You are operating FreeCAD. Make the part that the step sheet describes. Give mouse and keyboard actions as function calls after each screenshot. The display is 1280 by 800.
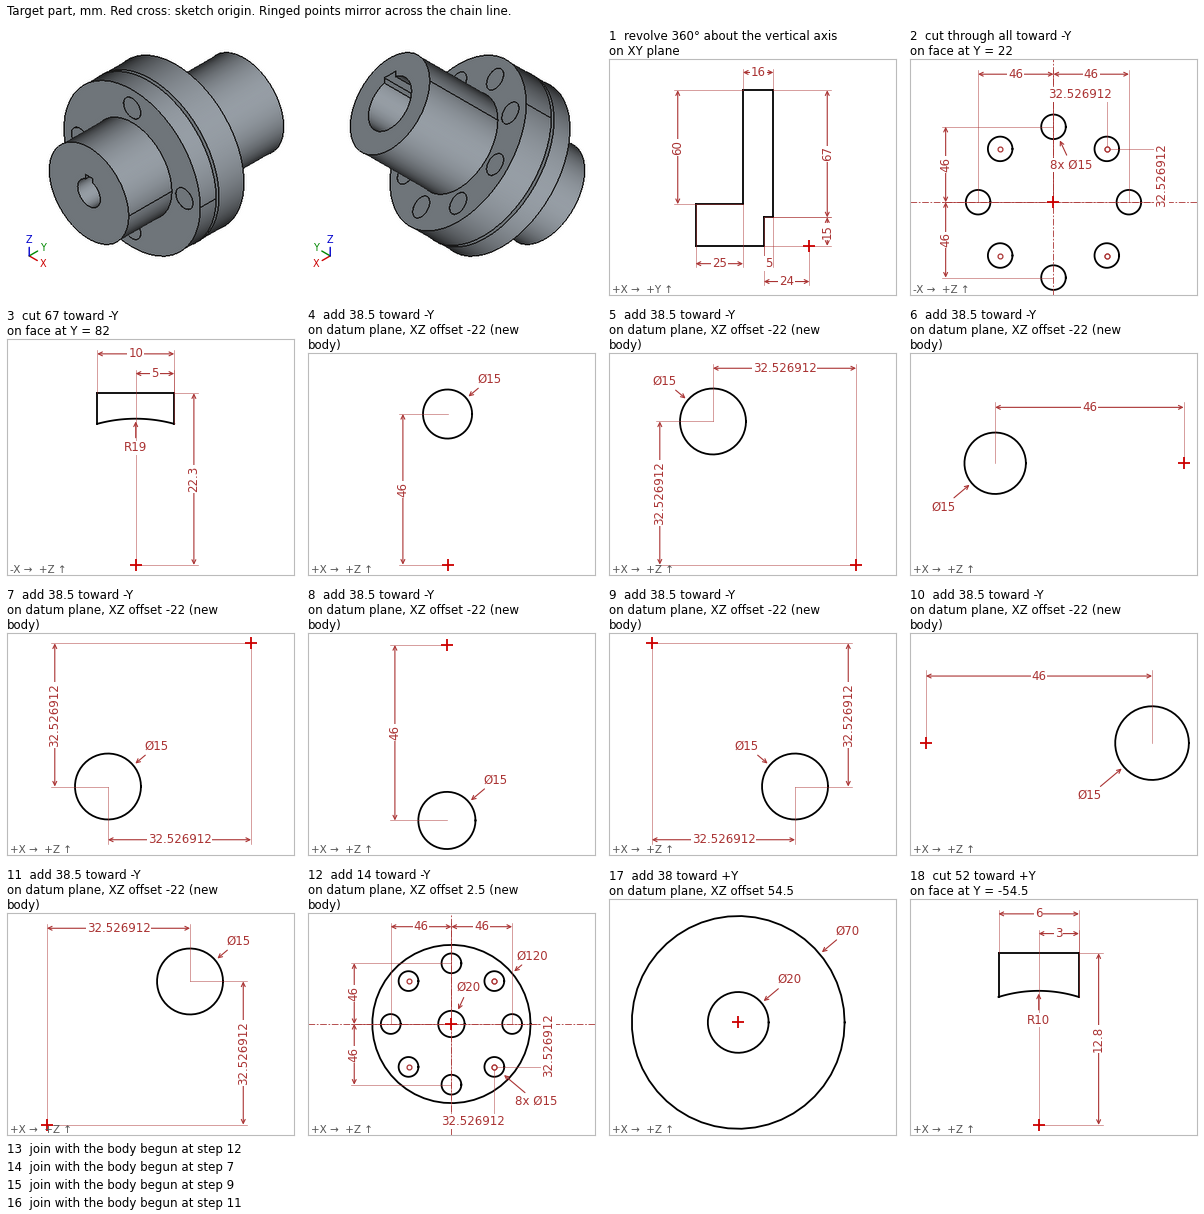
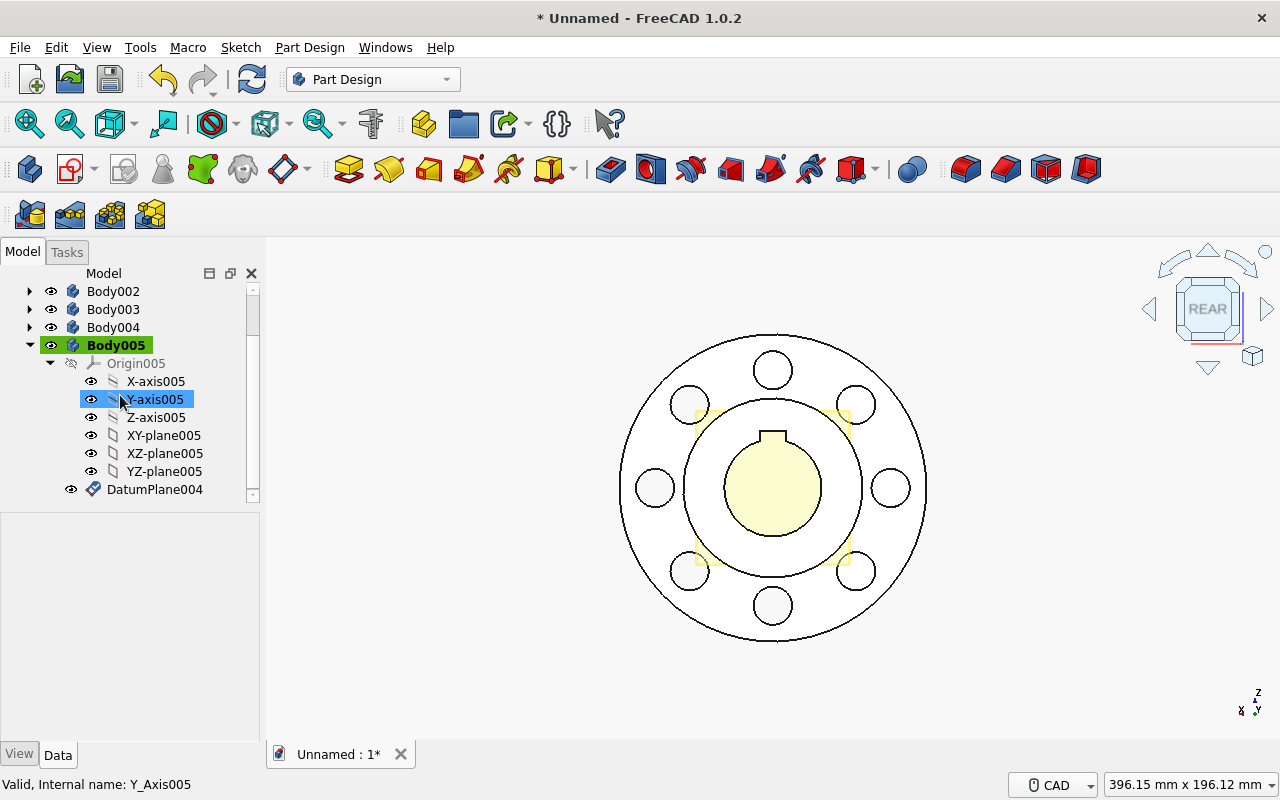
click(116, 489)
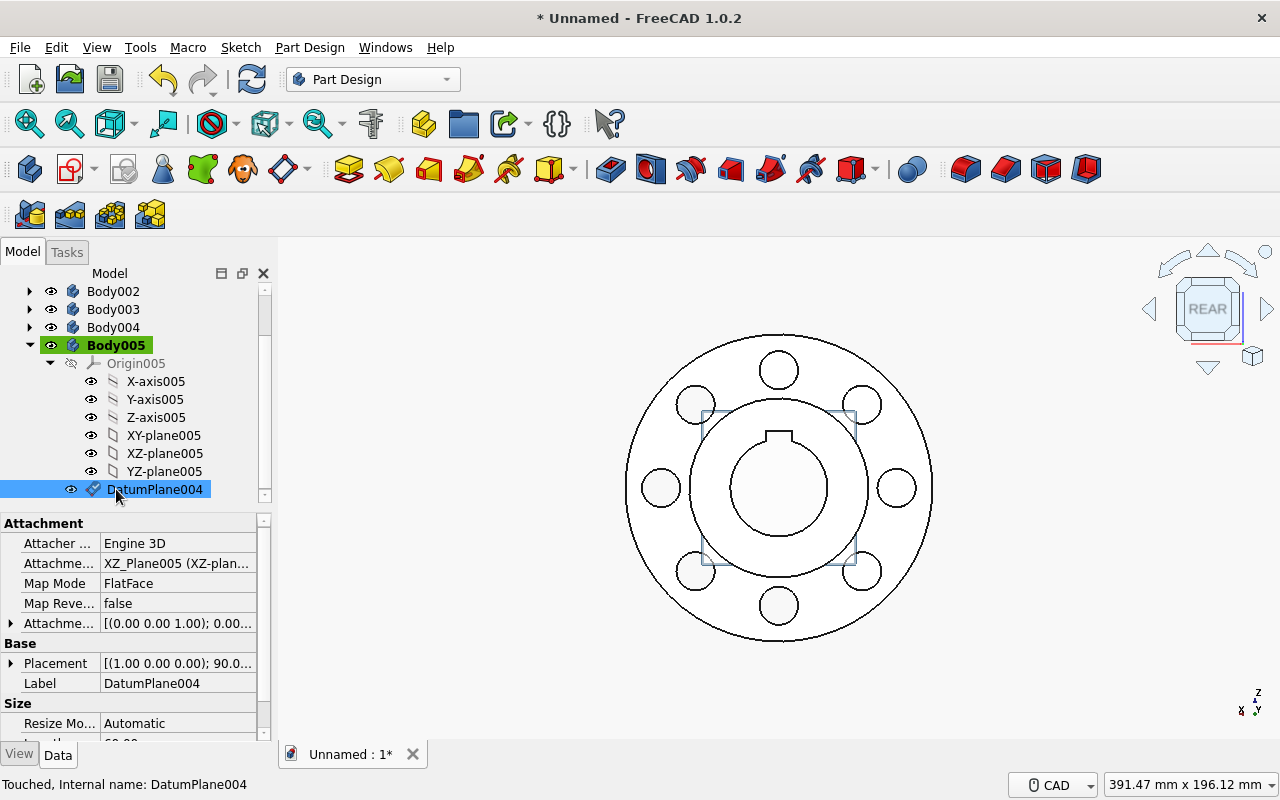
click(70, 170)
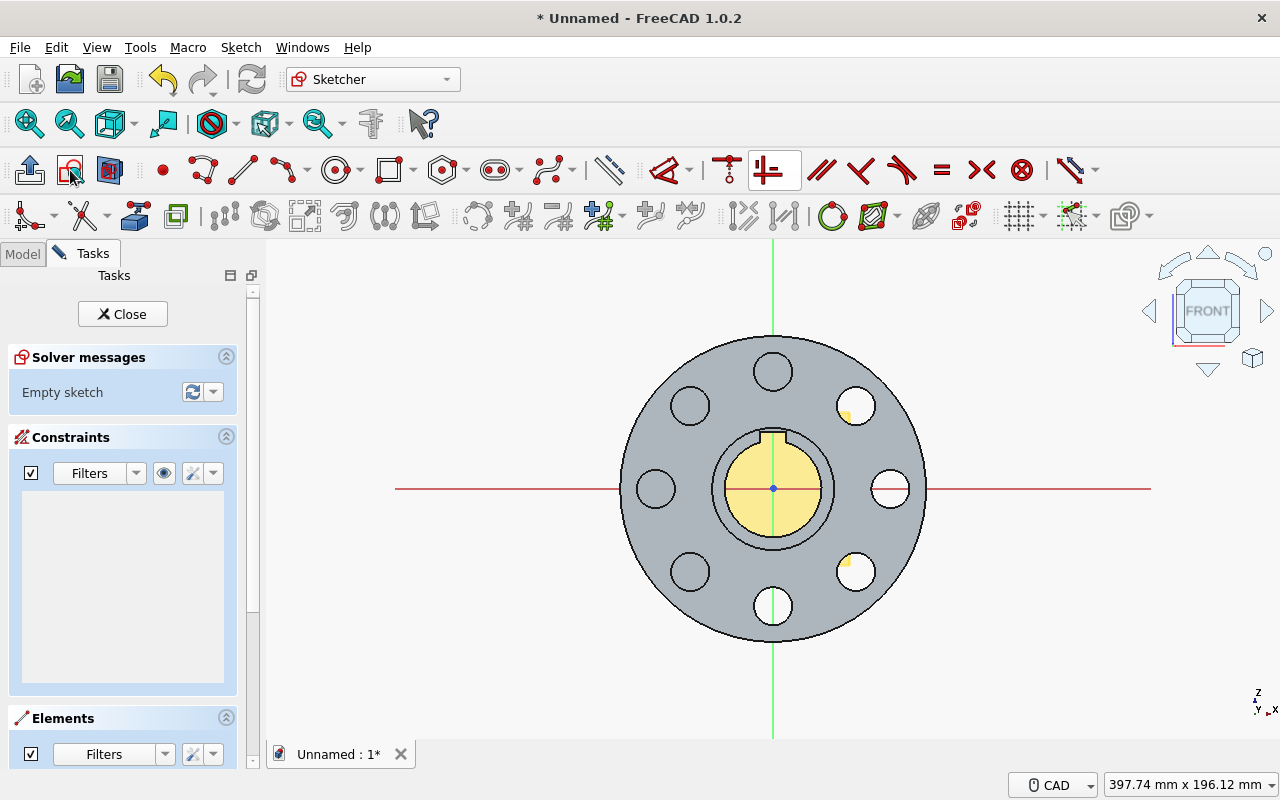
scroll(782, 621, up, 11)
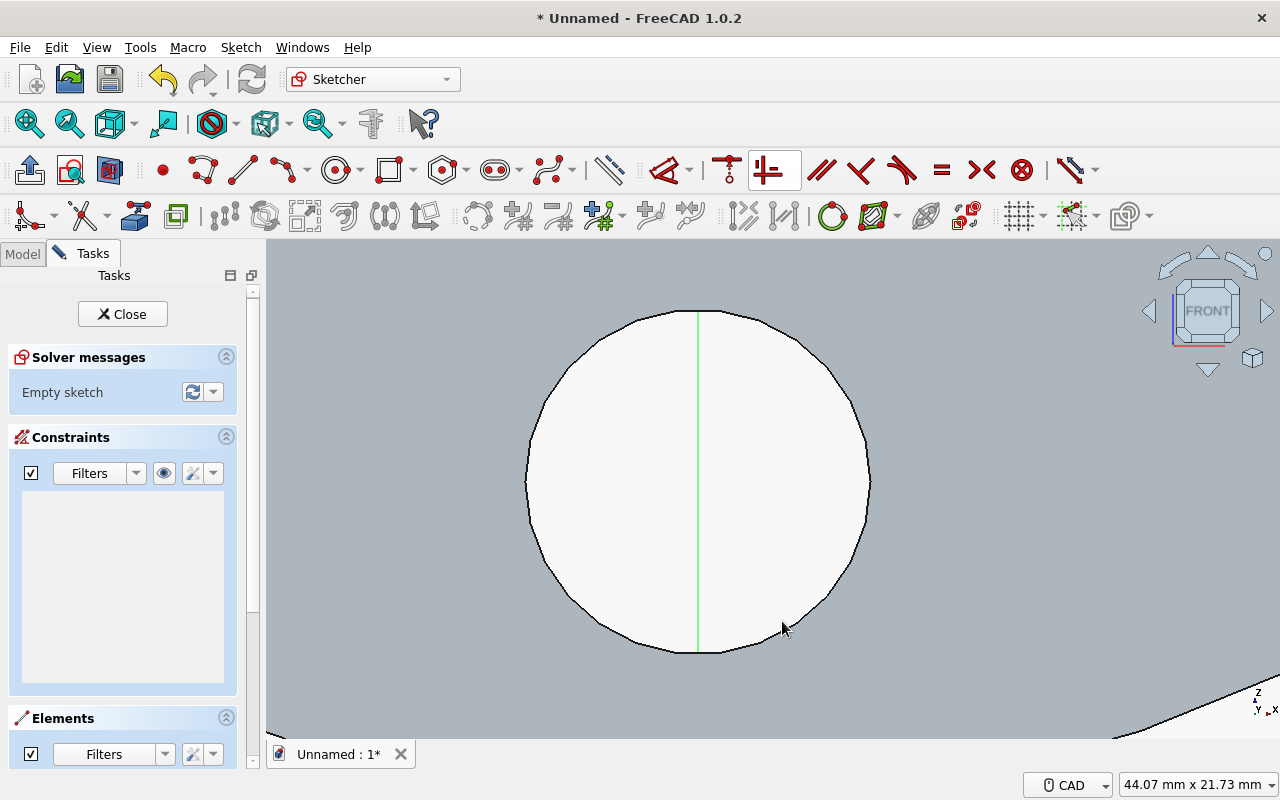
click(336, 170)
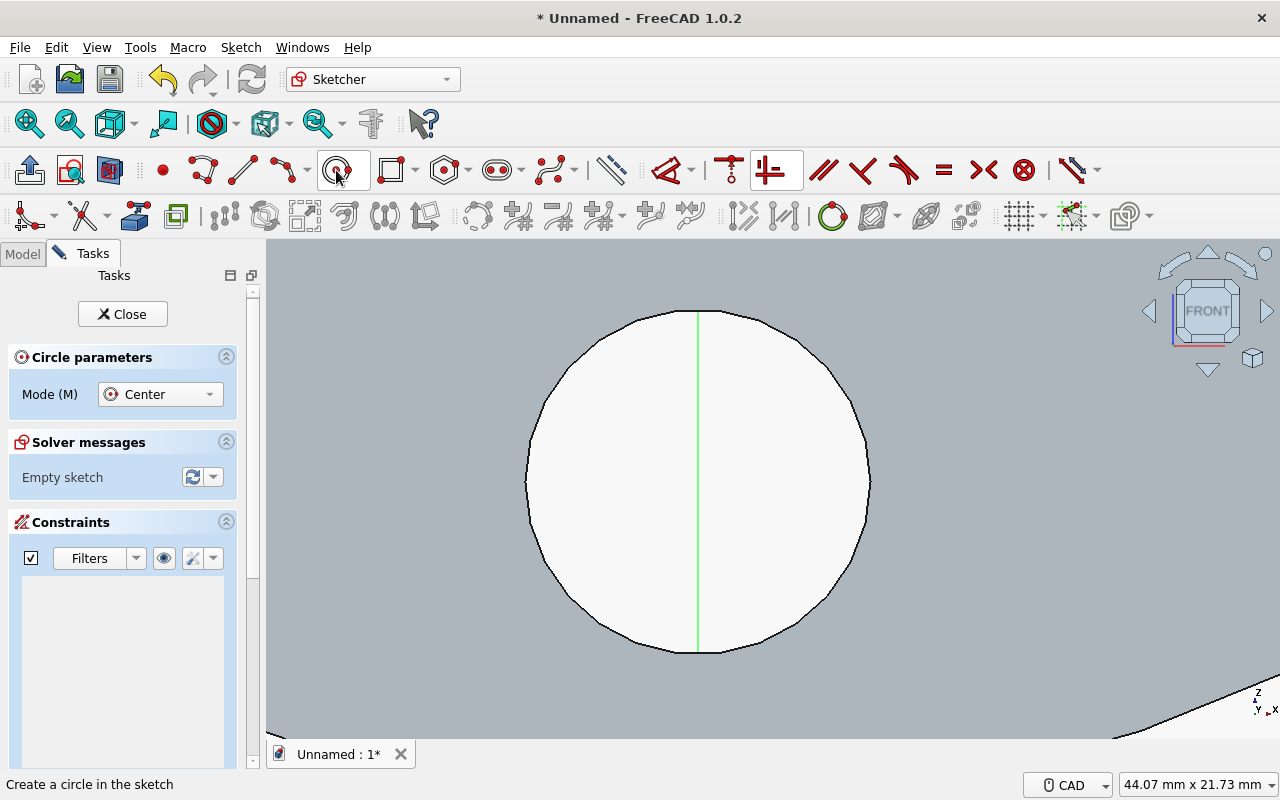
click(698, 482)
click(820, 360)
key(Escape)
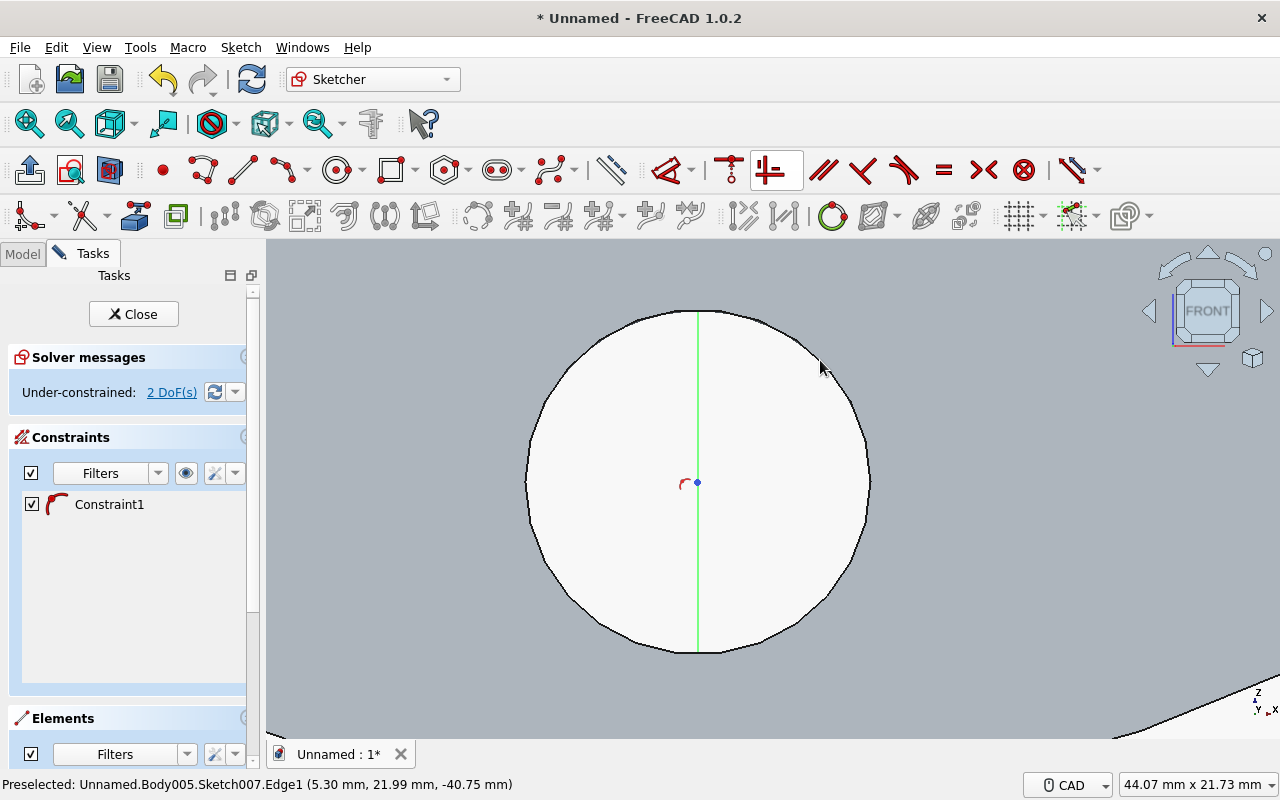
click(666, 170)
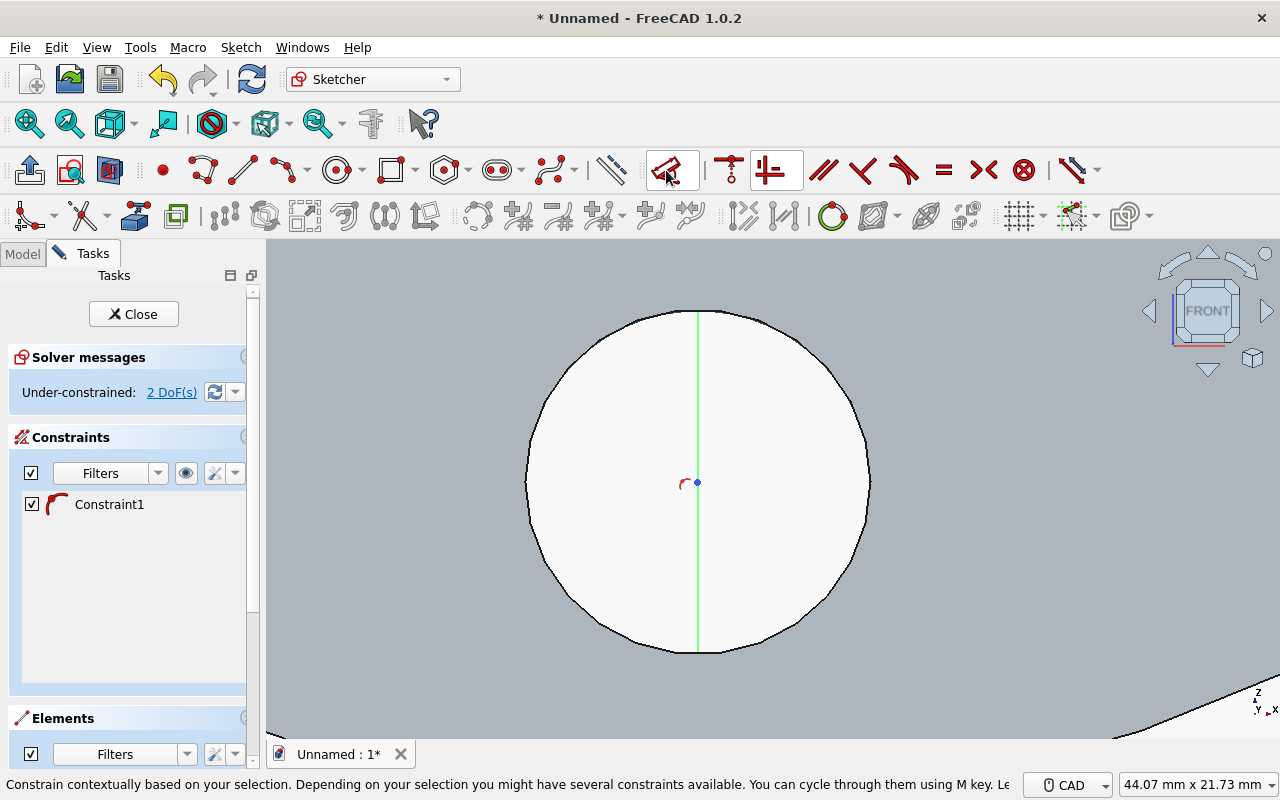
click(820, 361)
click(843, 338)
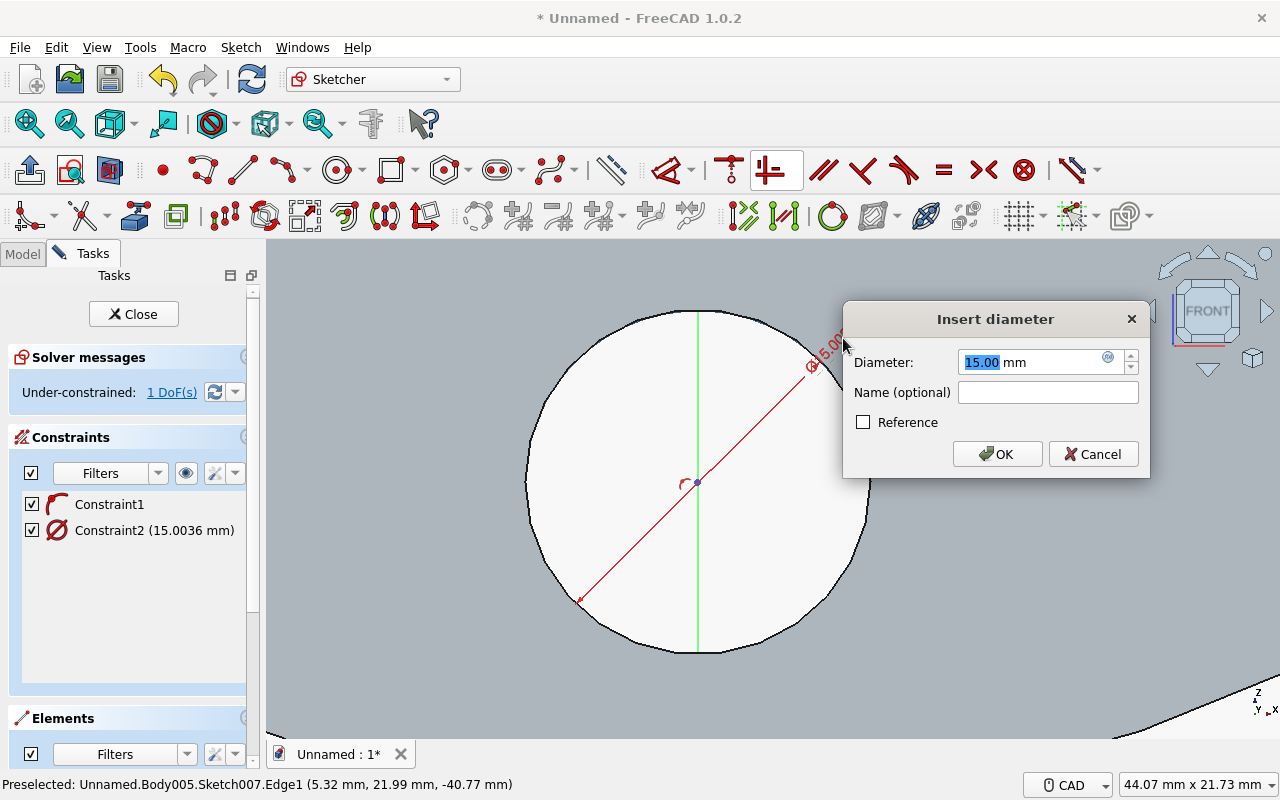
text(15)
key(Return)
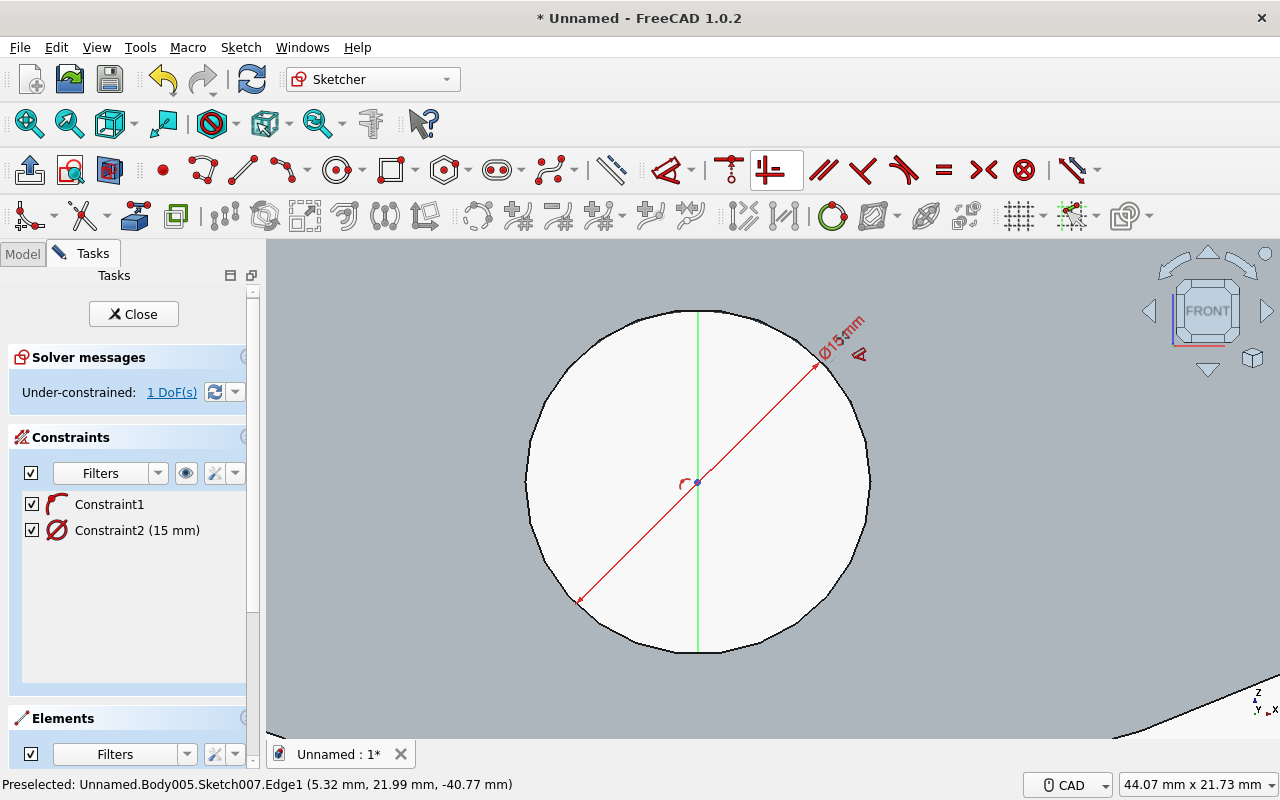
click(698, 483)
click(732, 375)